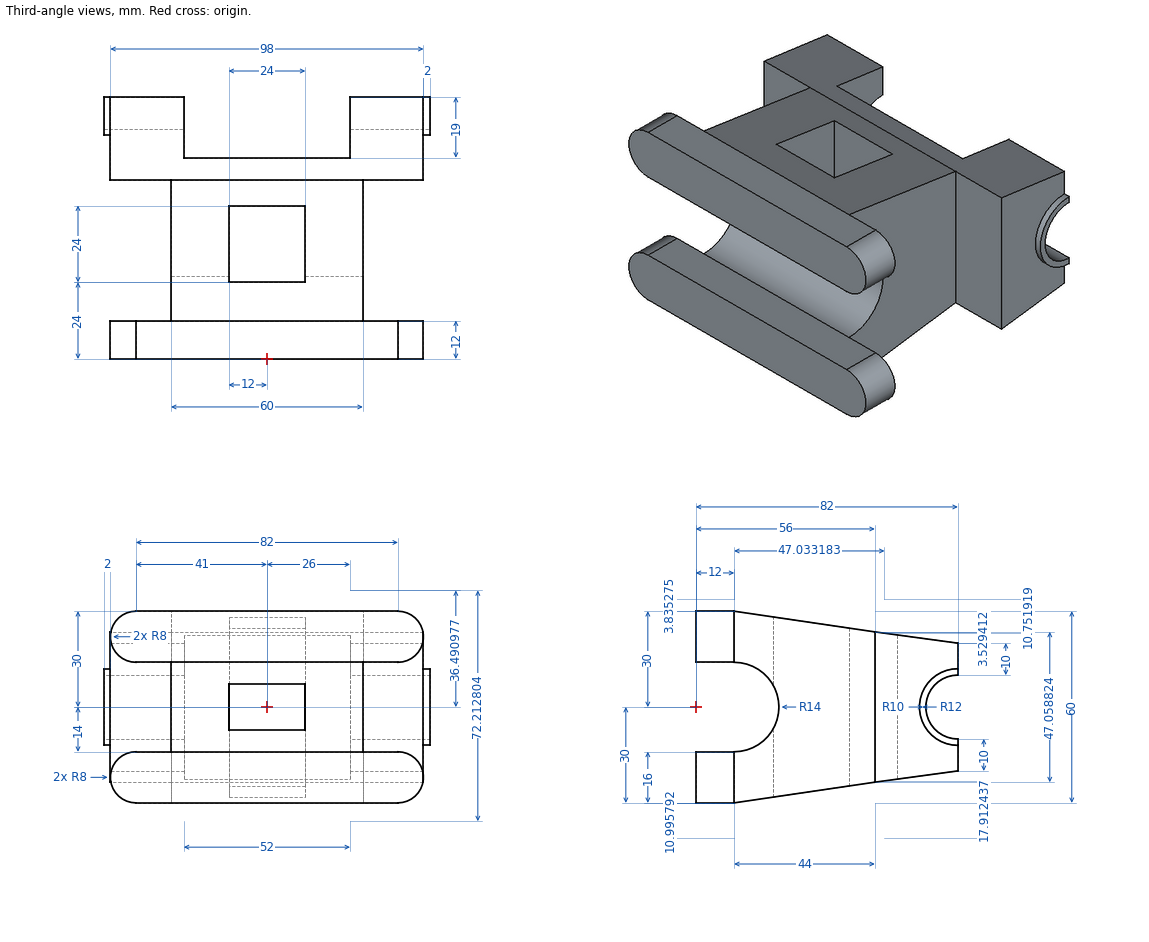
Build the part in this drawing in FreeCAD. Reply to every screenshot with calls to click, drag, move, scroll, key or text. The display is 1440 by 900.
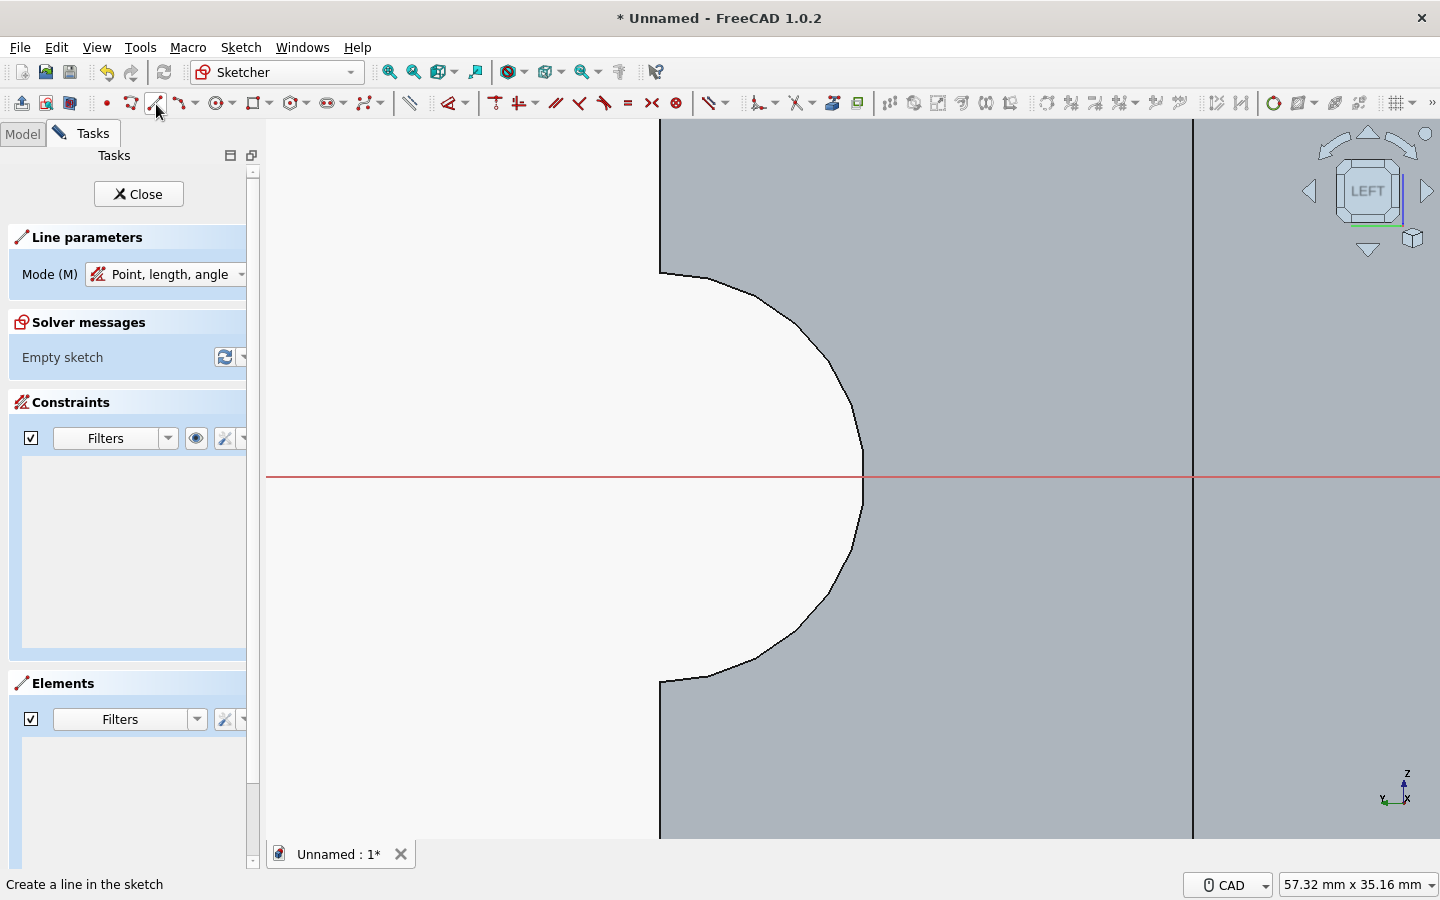
click(660, 232)
click(660, 273)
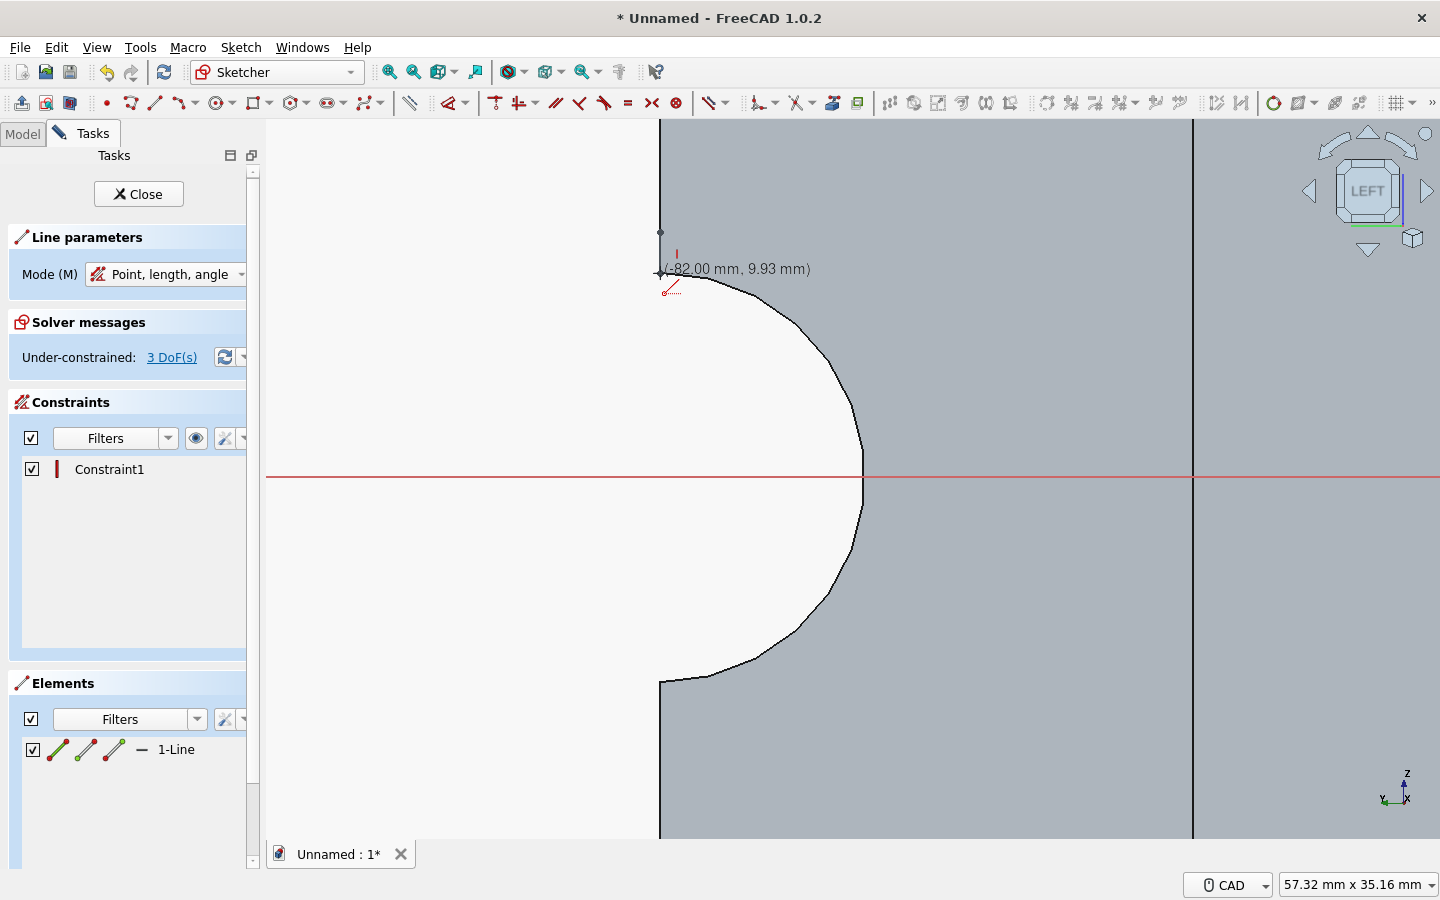
click(660, 682)
click(660, 723)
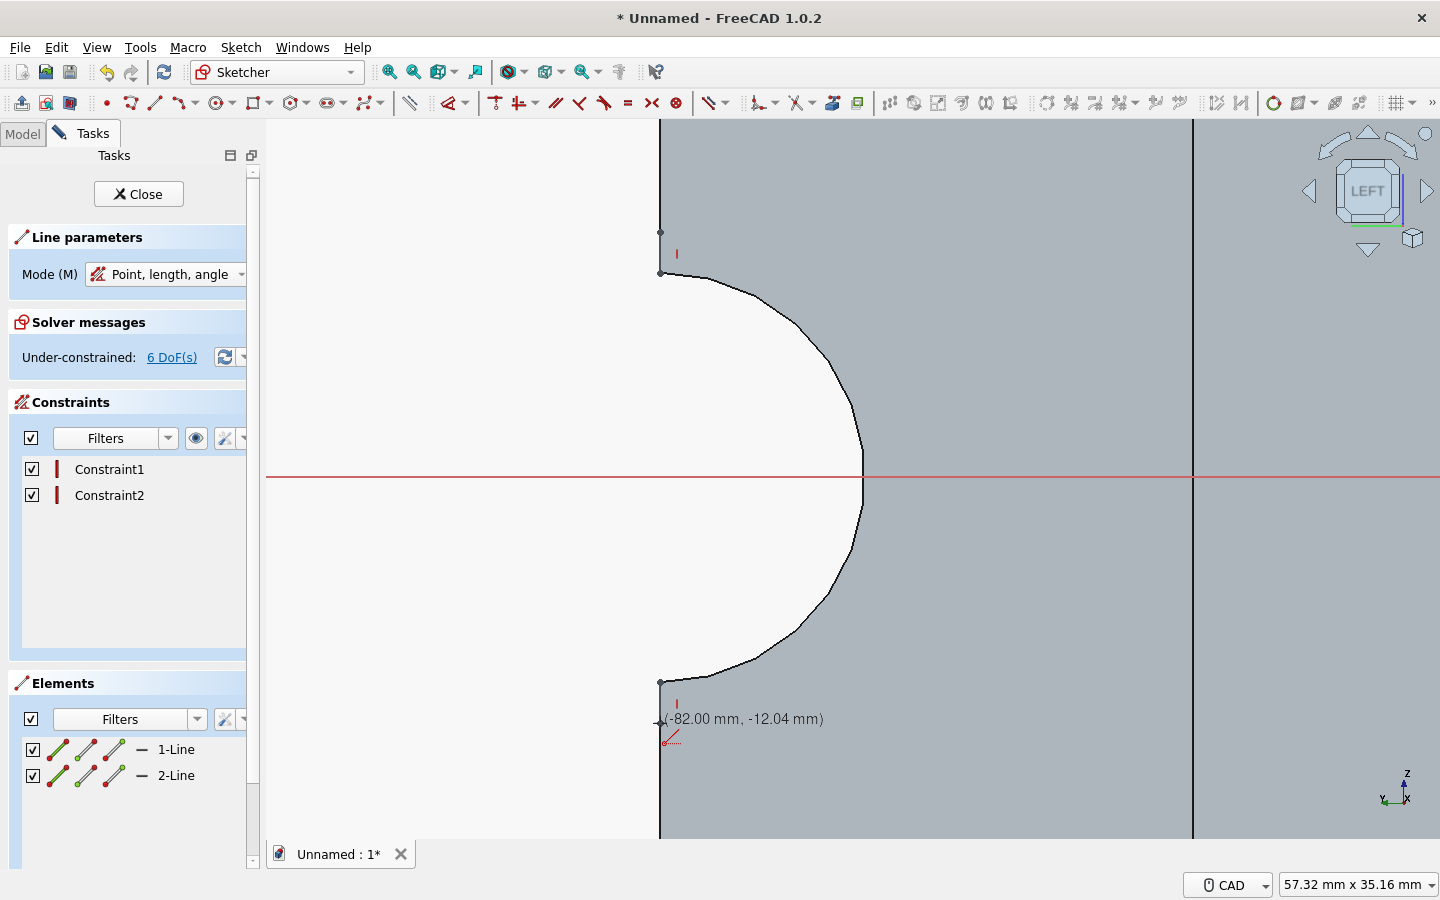
click(180, 104)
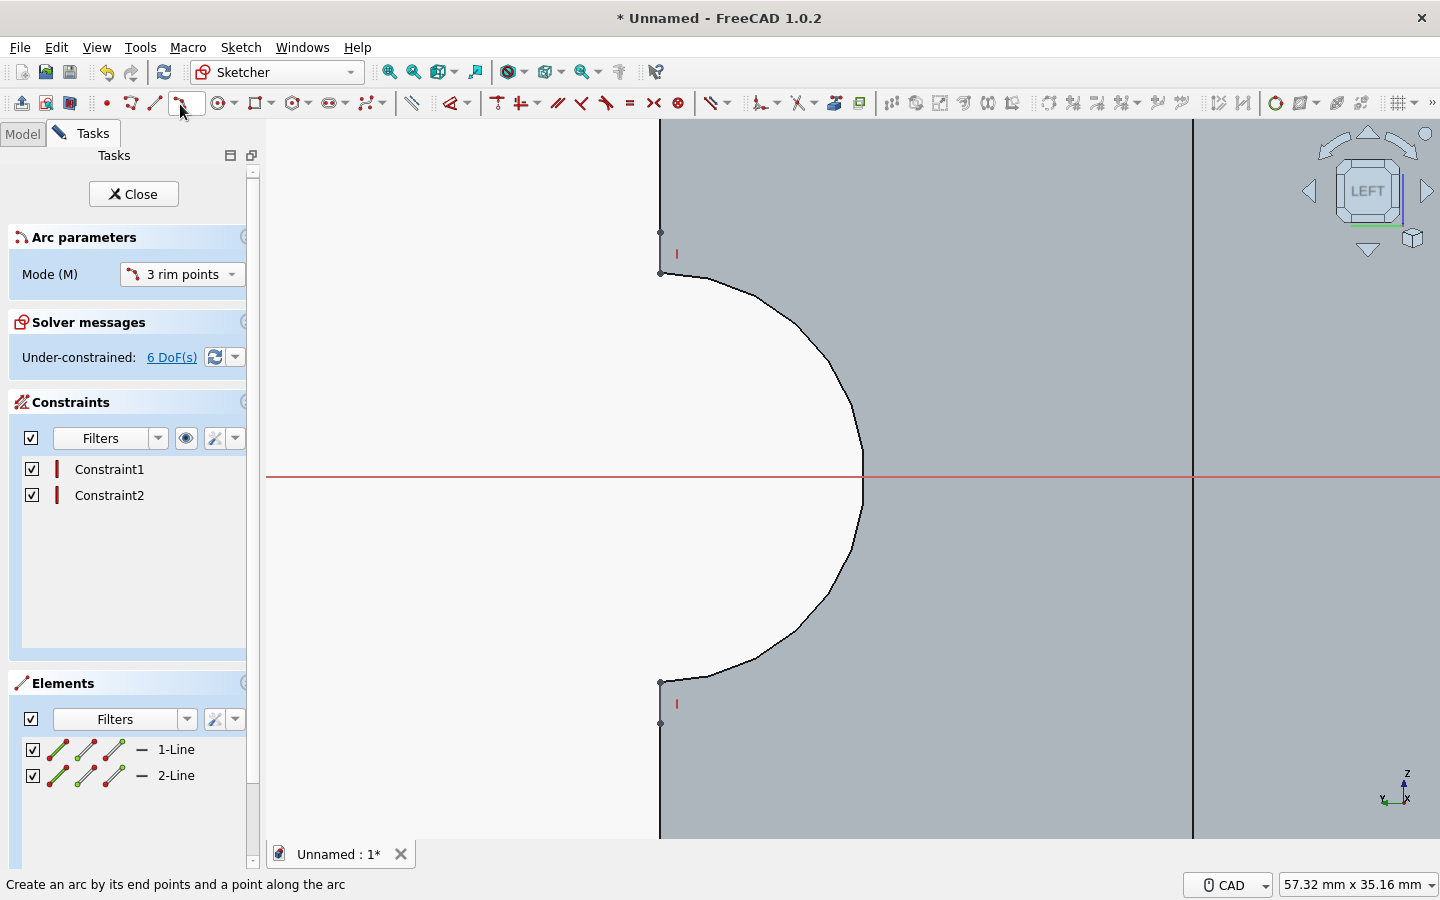
click(660, 274)
click(660, 683)
click(855, 541)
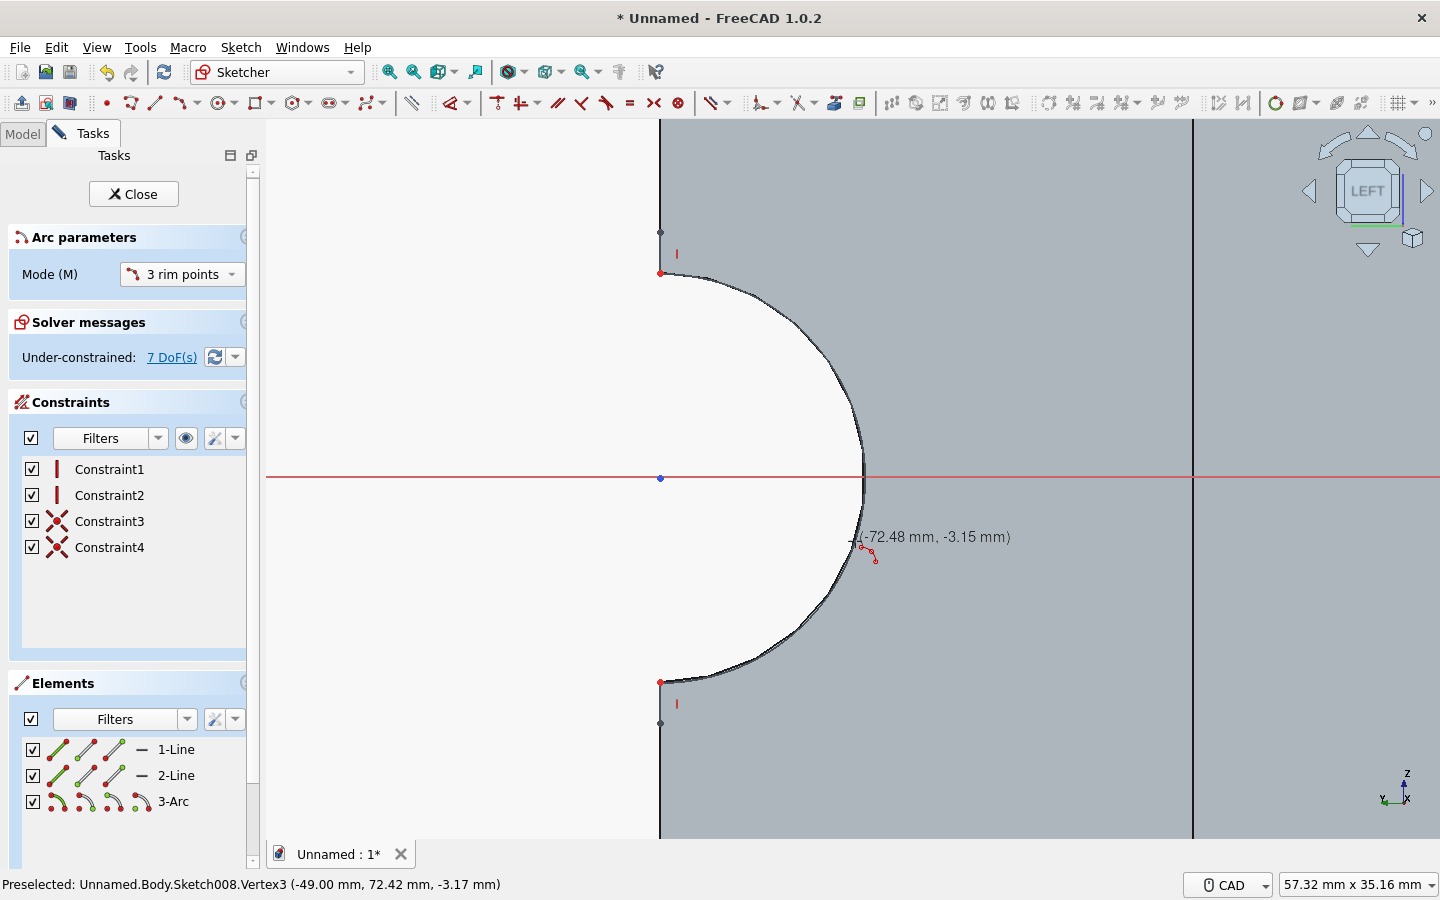
click(660, 724)
click(660, 233)
click(894, 553)
key(Escape)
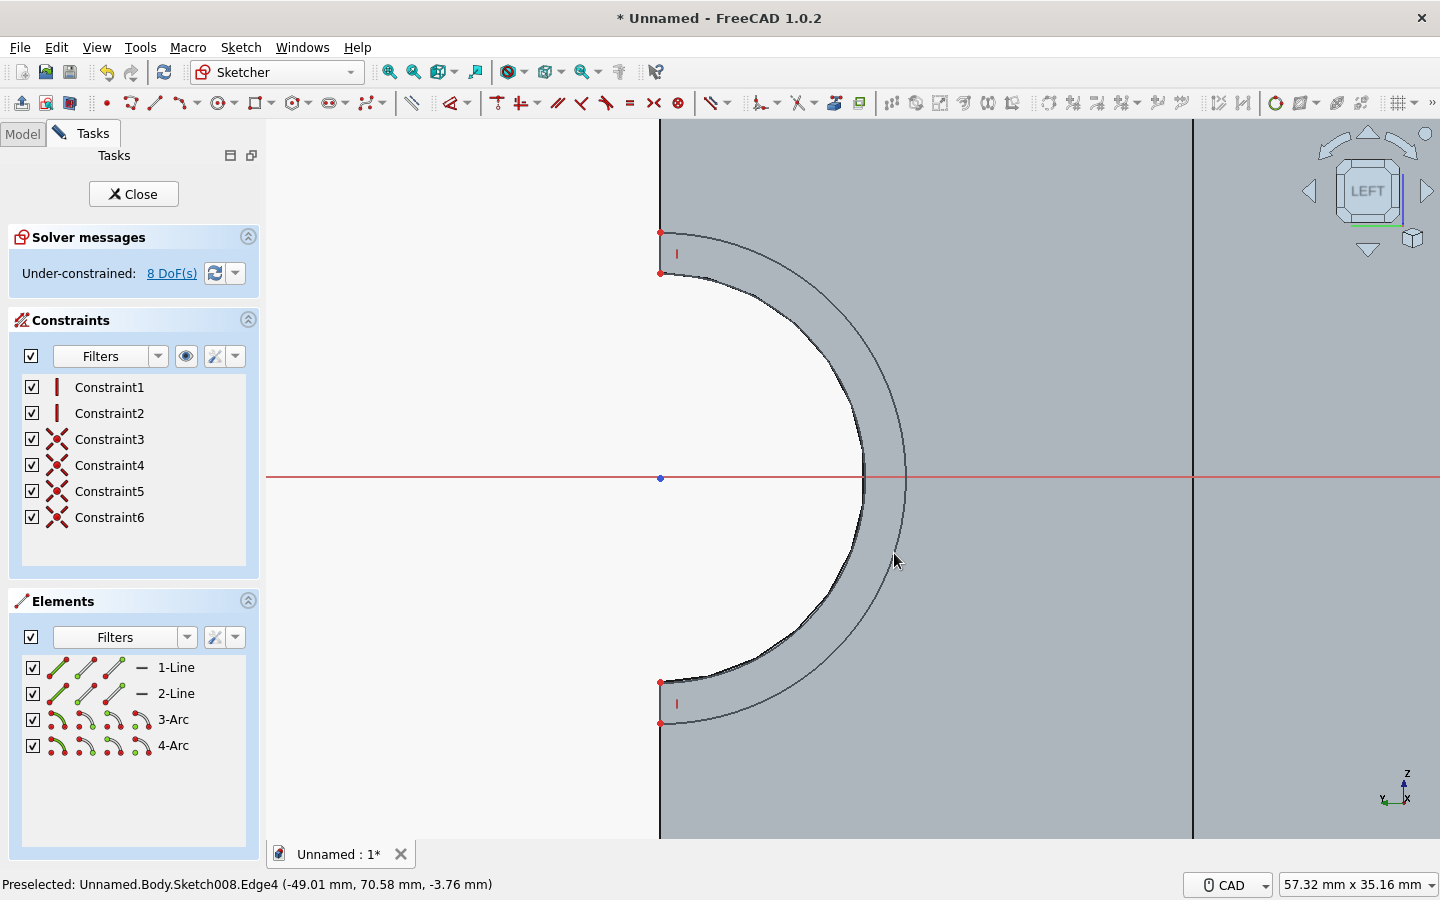
click(826, 599)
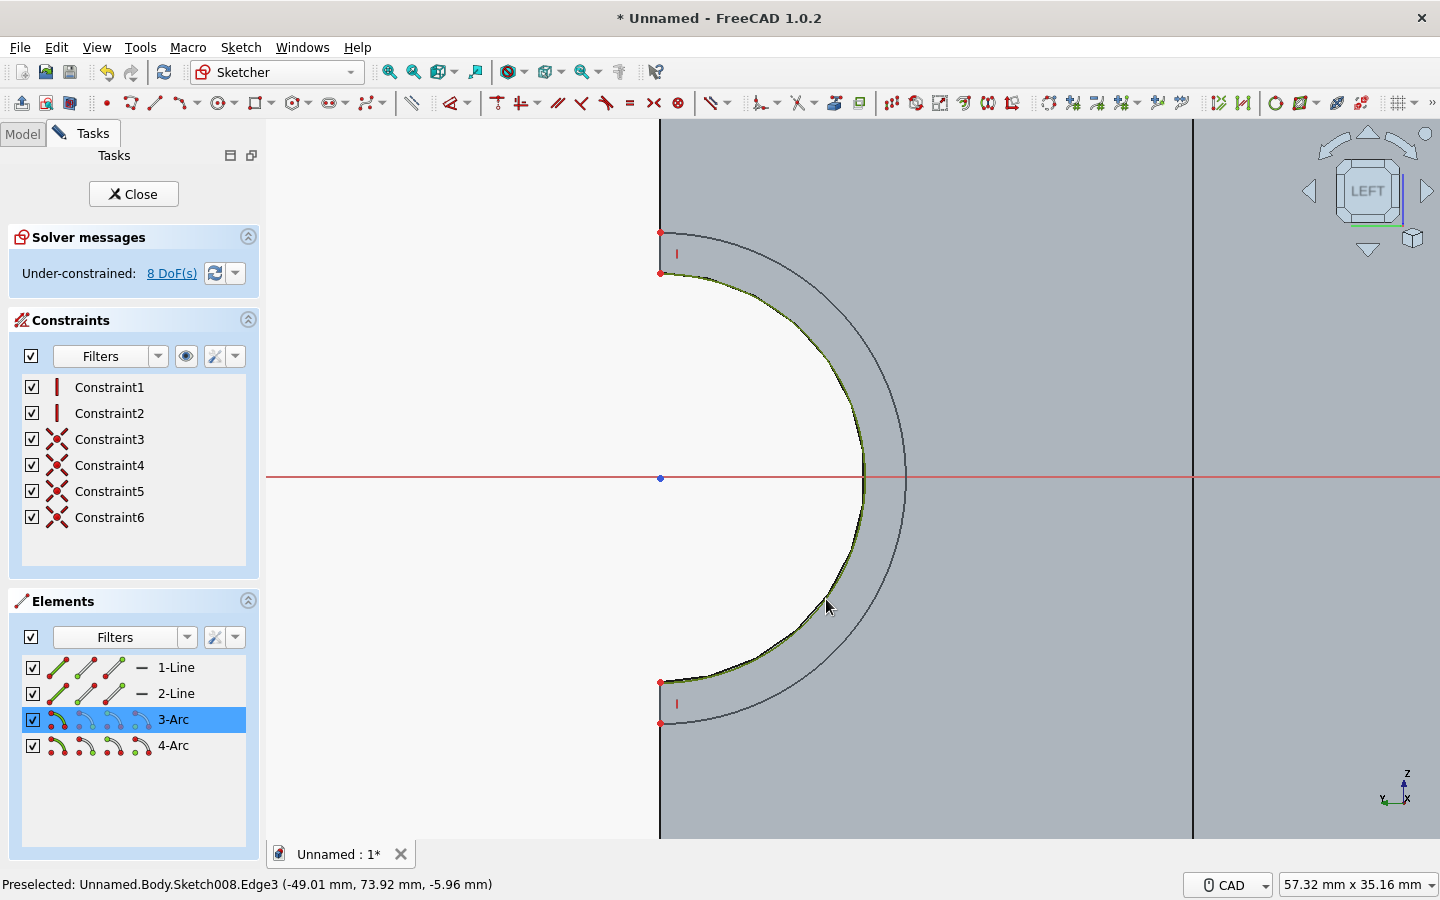
click(859, 623)